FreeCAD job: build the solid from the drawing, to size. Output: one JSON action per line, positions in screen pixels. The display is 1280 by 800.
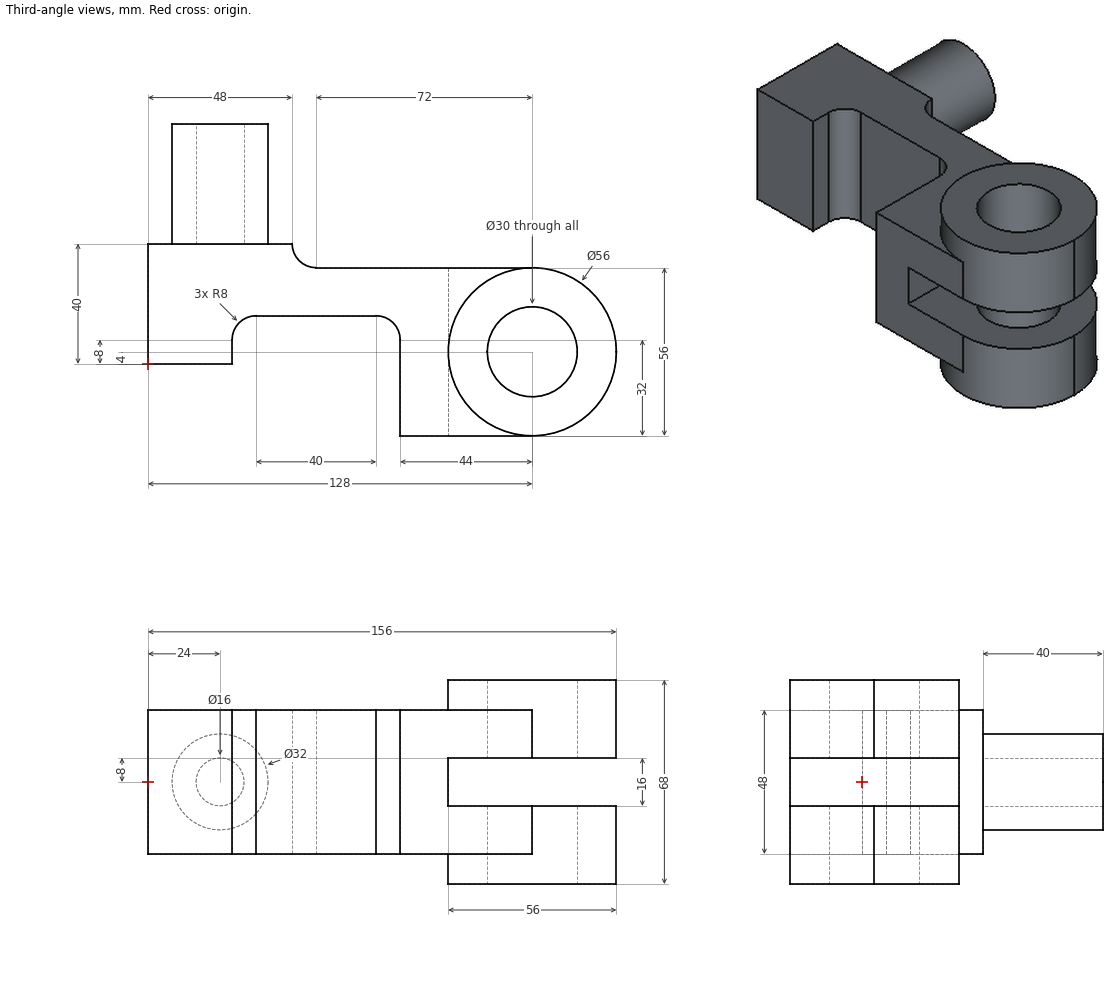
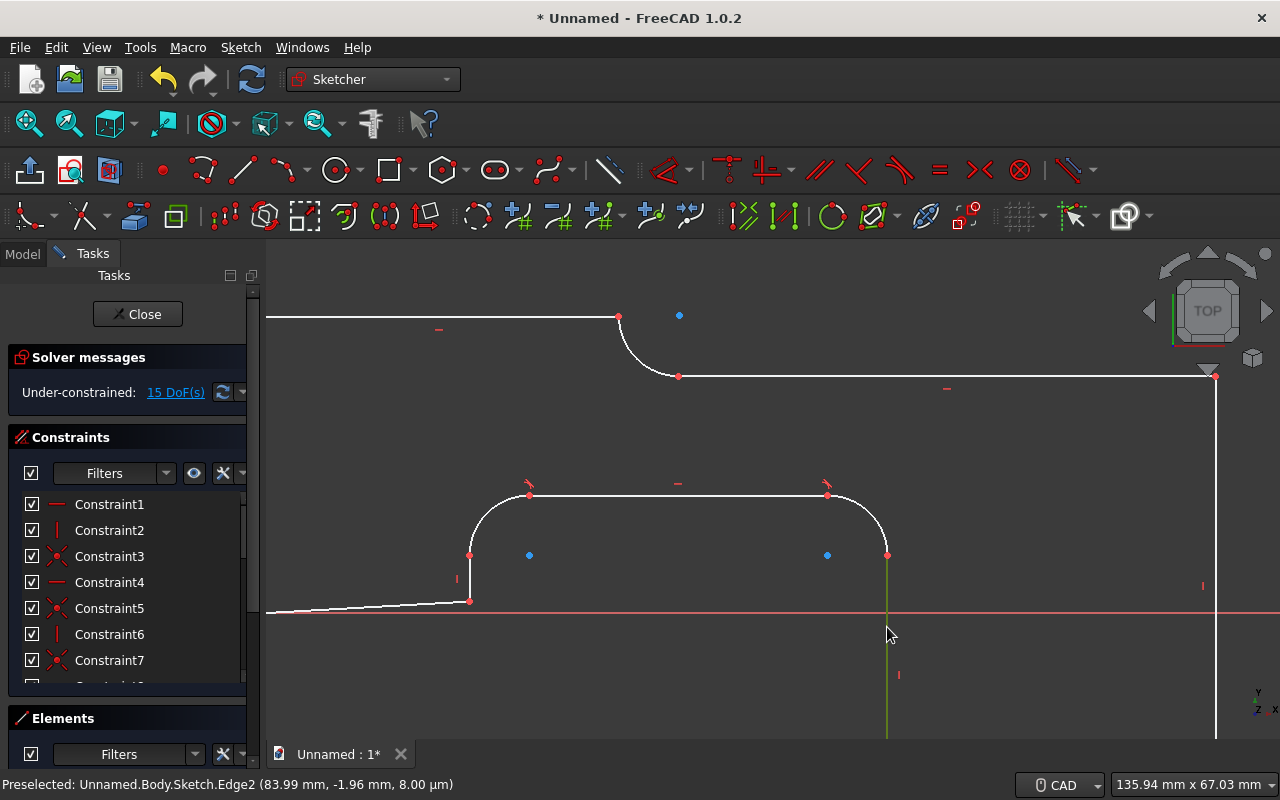
{"action": "left_click", "coordinate": [881, 528]}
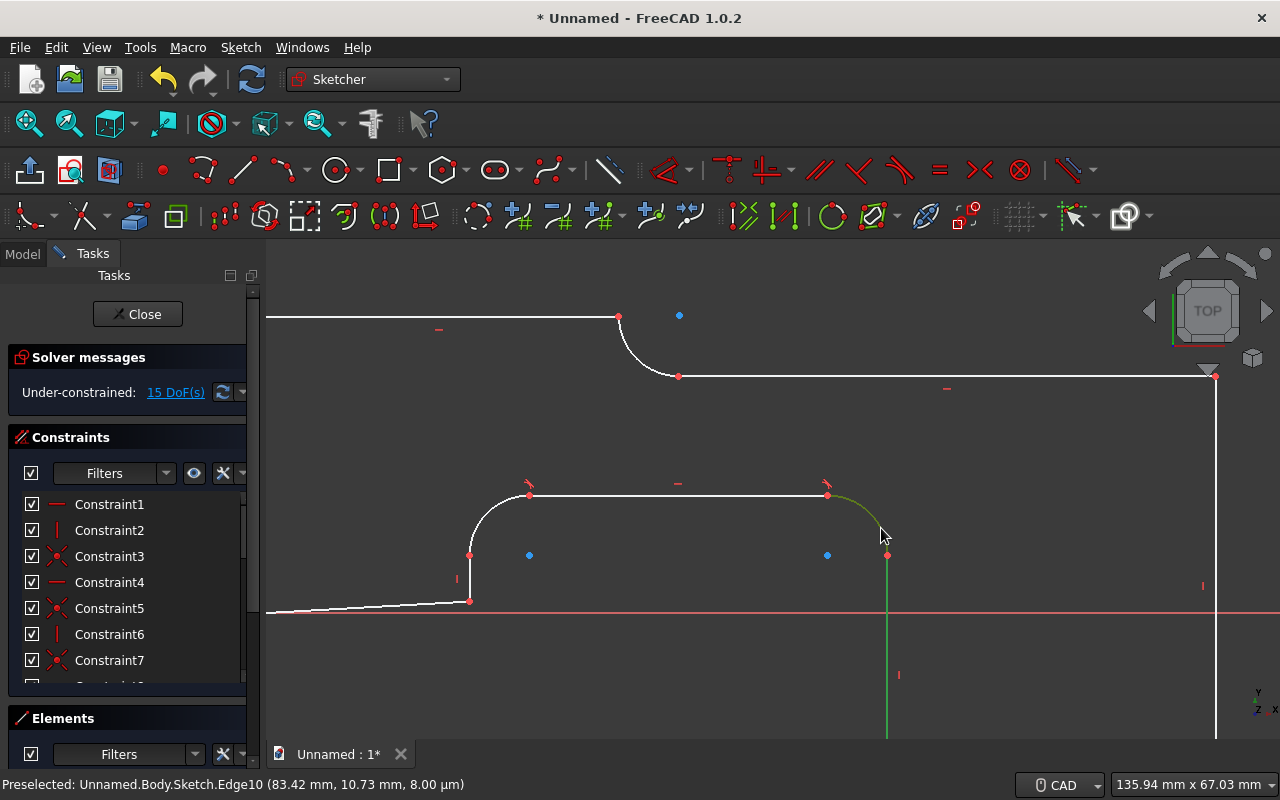
{"action": "left_click", "coordinate": [900, 170]}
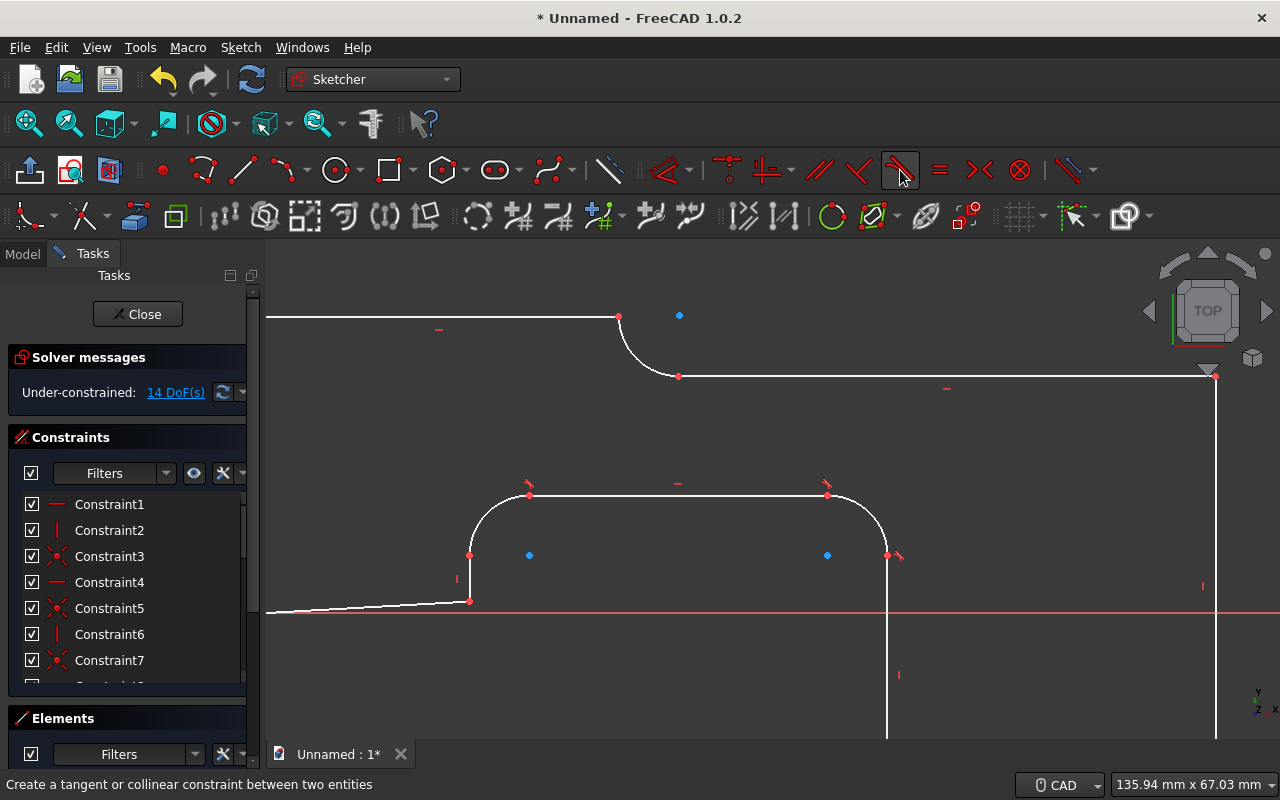
{"action": "left_click", "coordinate": [1055, 376]}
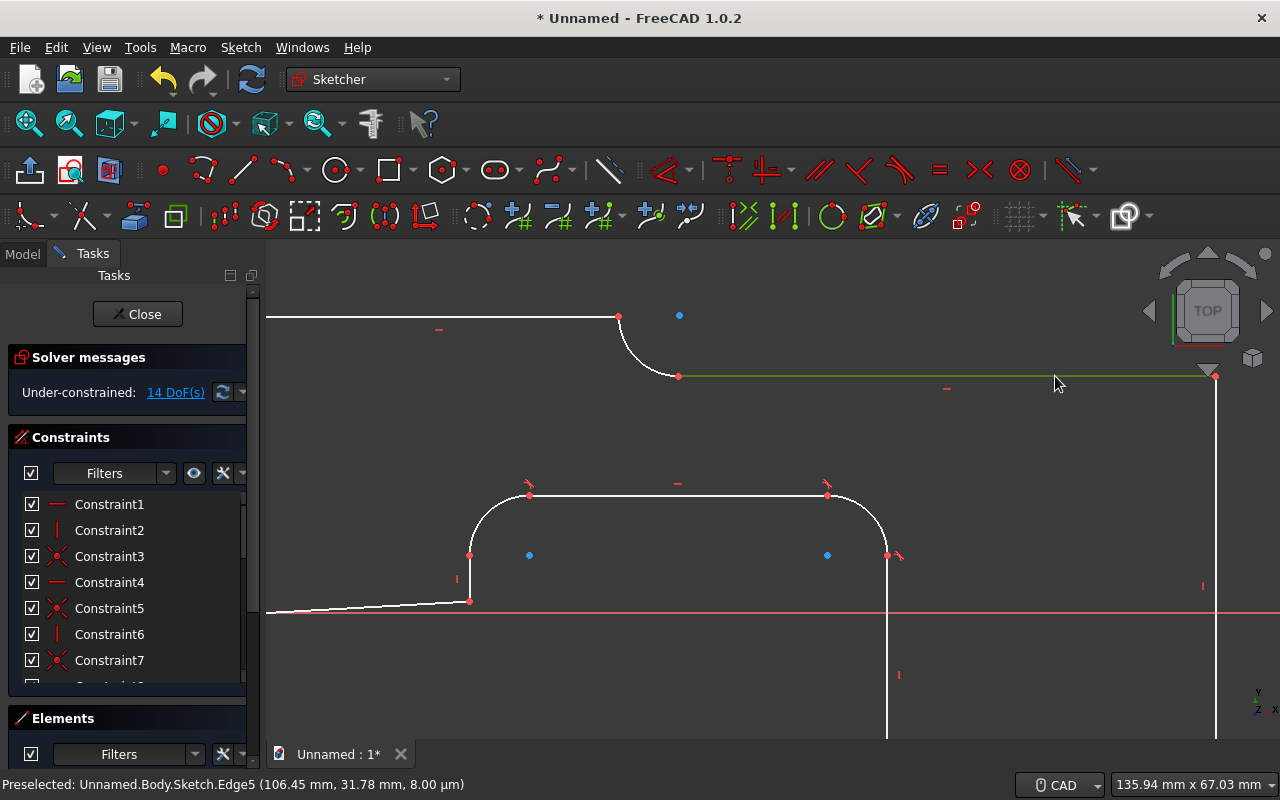
{"action": "left_click", "coordinate": [626, 344]}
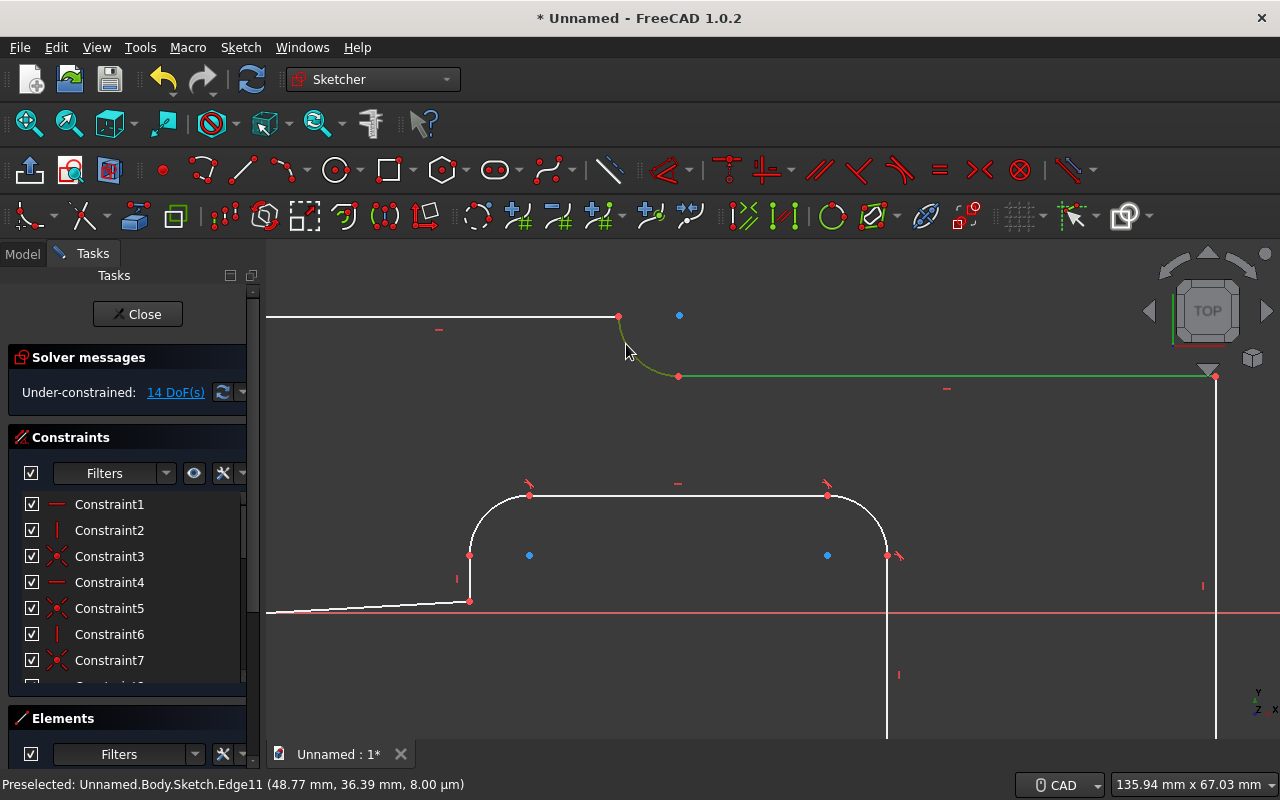
{"action": "left_click", "coordinate": [900, 170]}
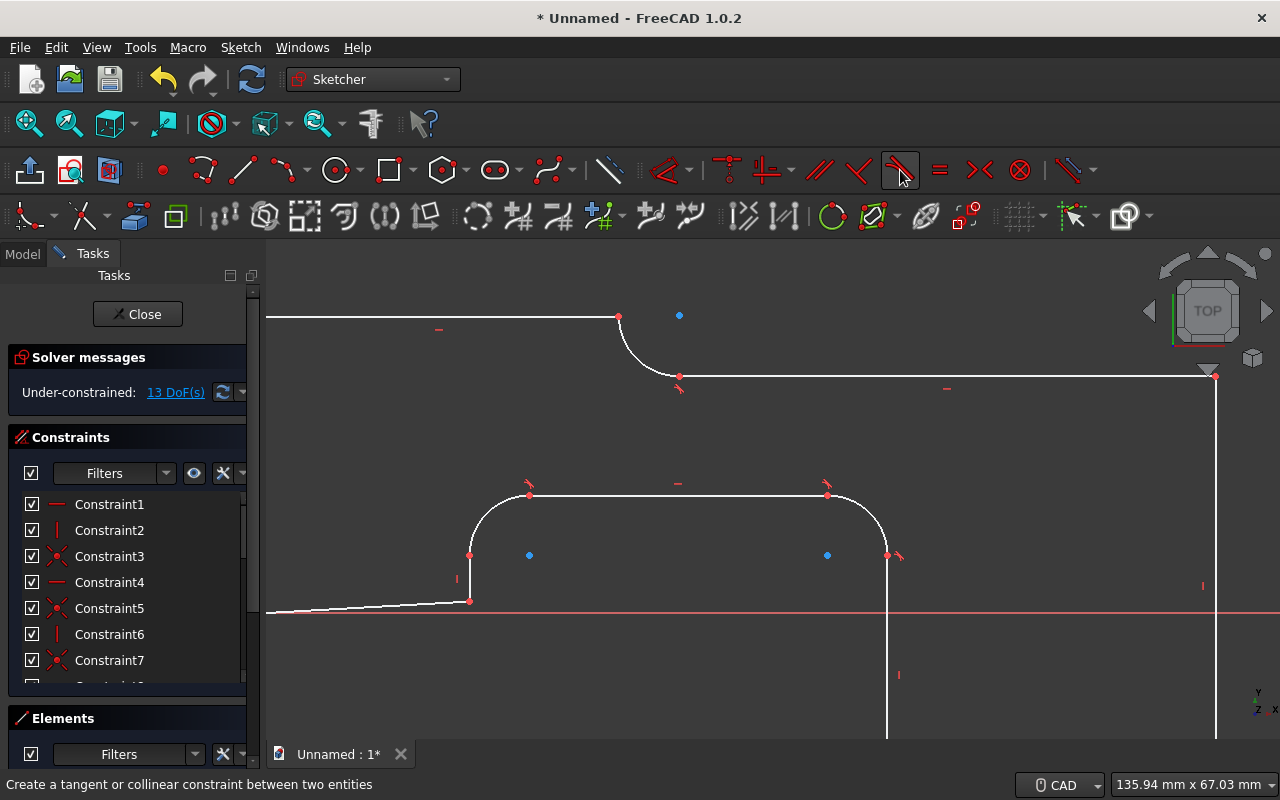
{"action": "left_click", "coordinate": [470, 588]}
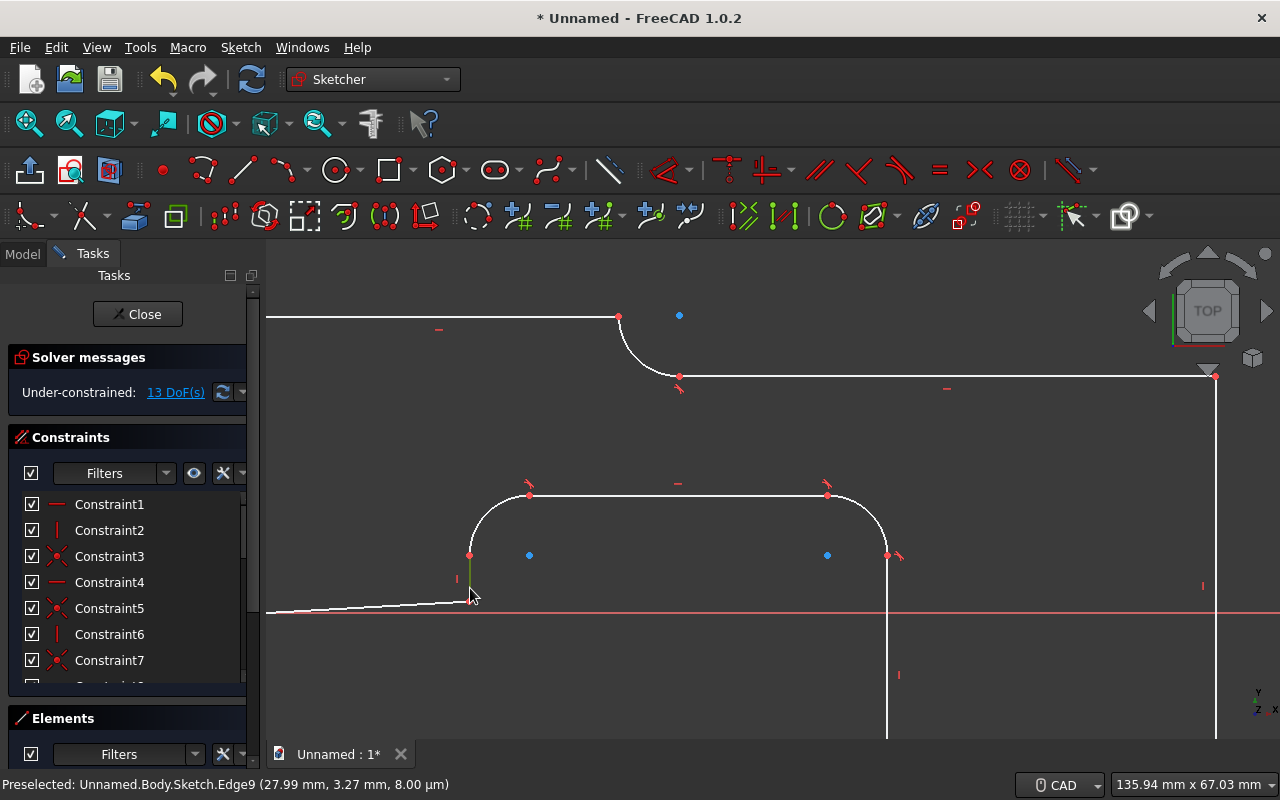
{"action": "left_click", "coordinate": [502, 502]}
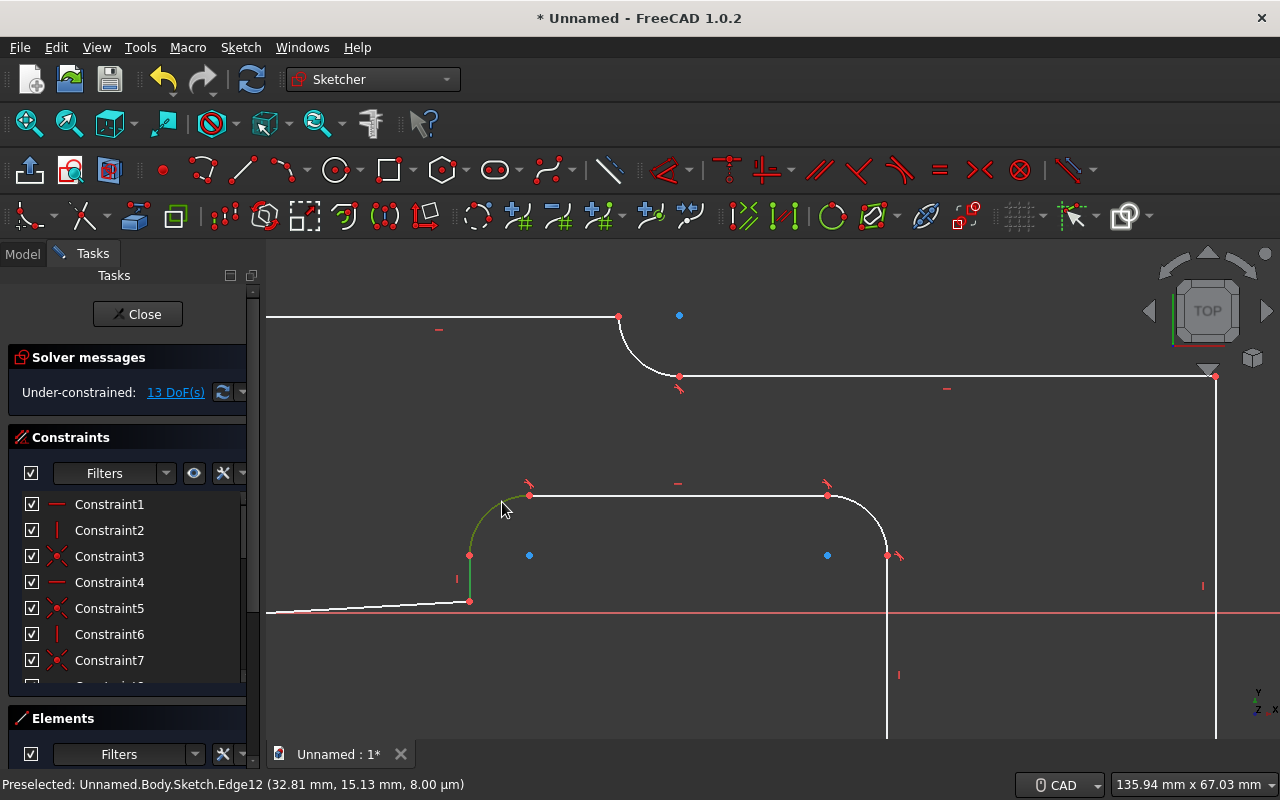
{"action": "key", "text": "t"}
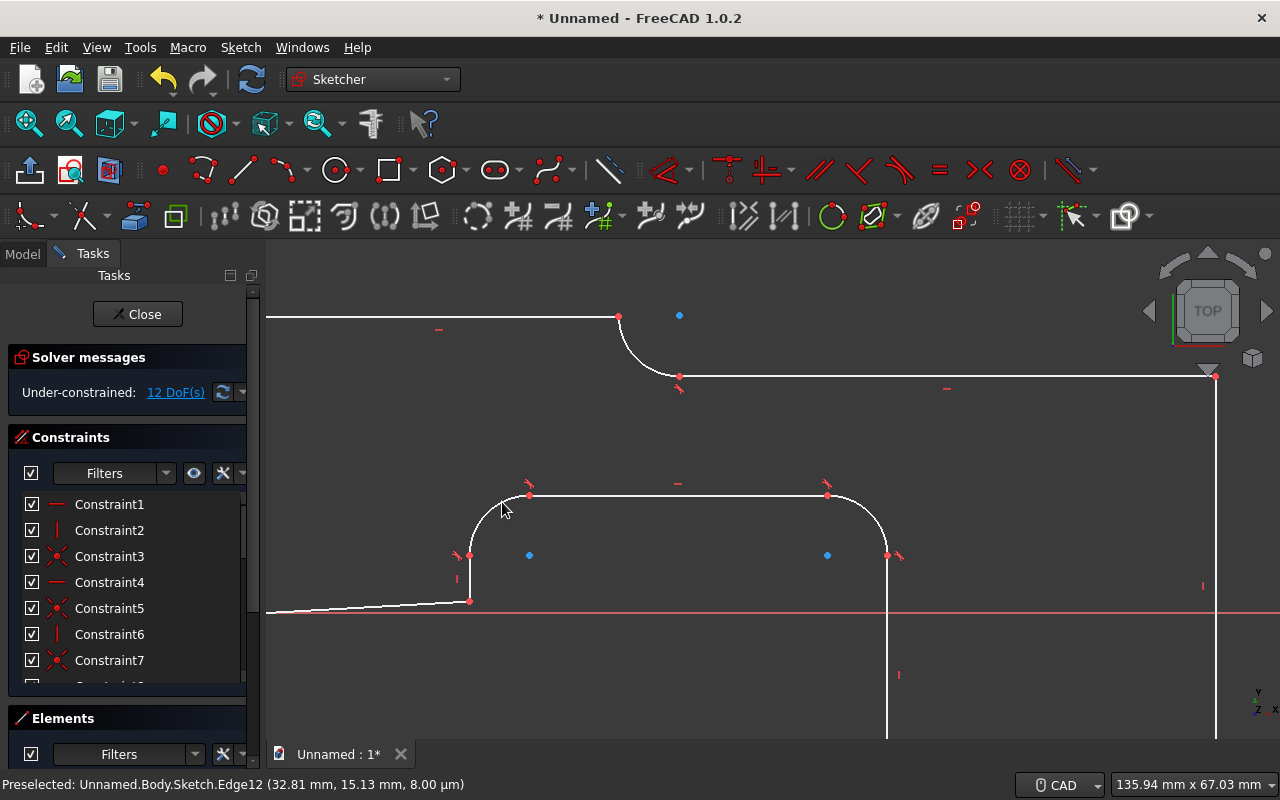
{"action": "left_click", "coordinate": [324, 610]}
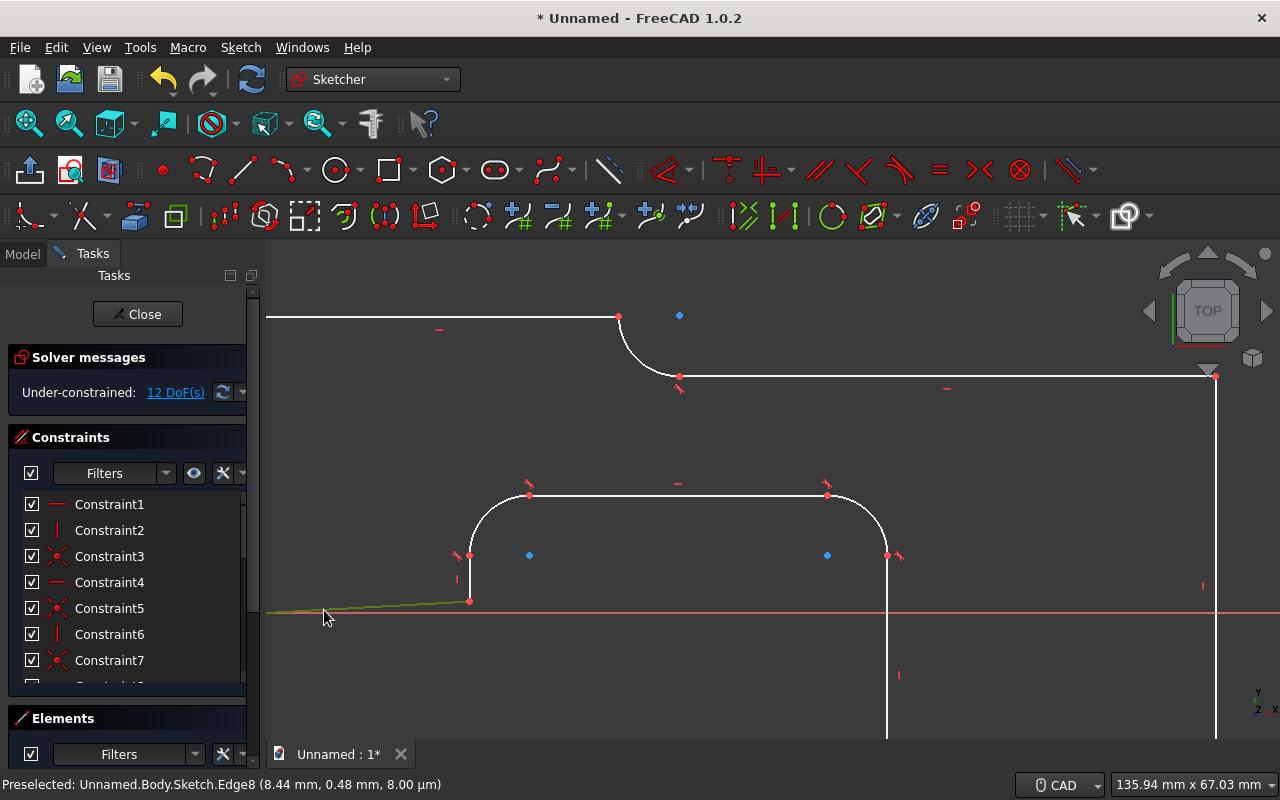
{"action": "left_click", "coordinate": [794, 170]}